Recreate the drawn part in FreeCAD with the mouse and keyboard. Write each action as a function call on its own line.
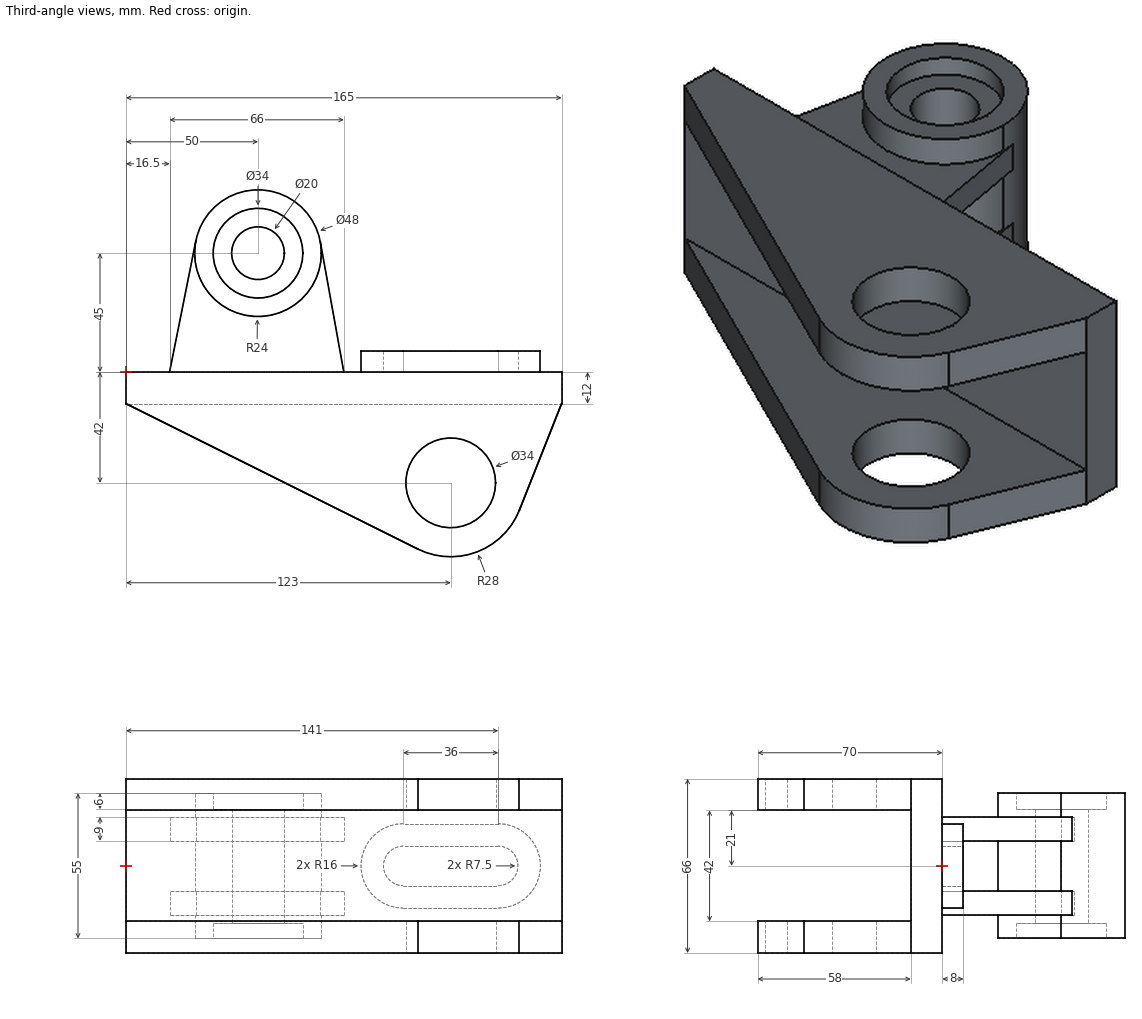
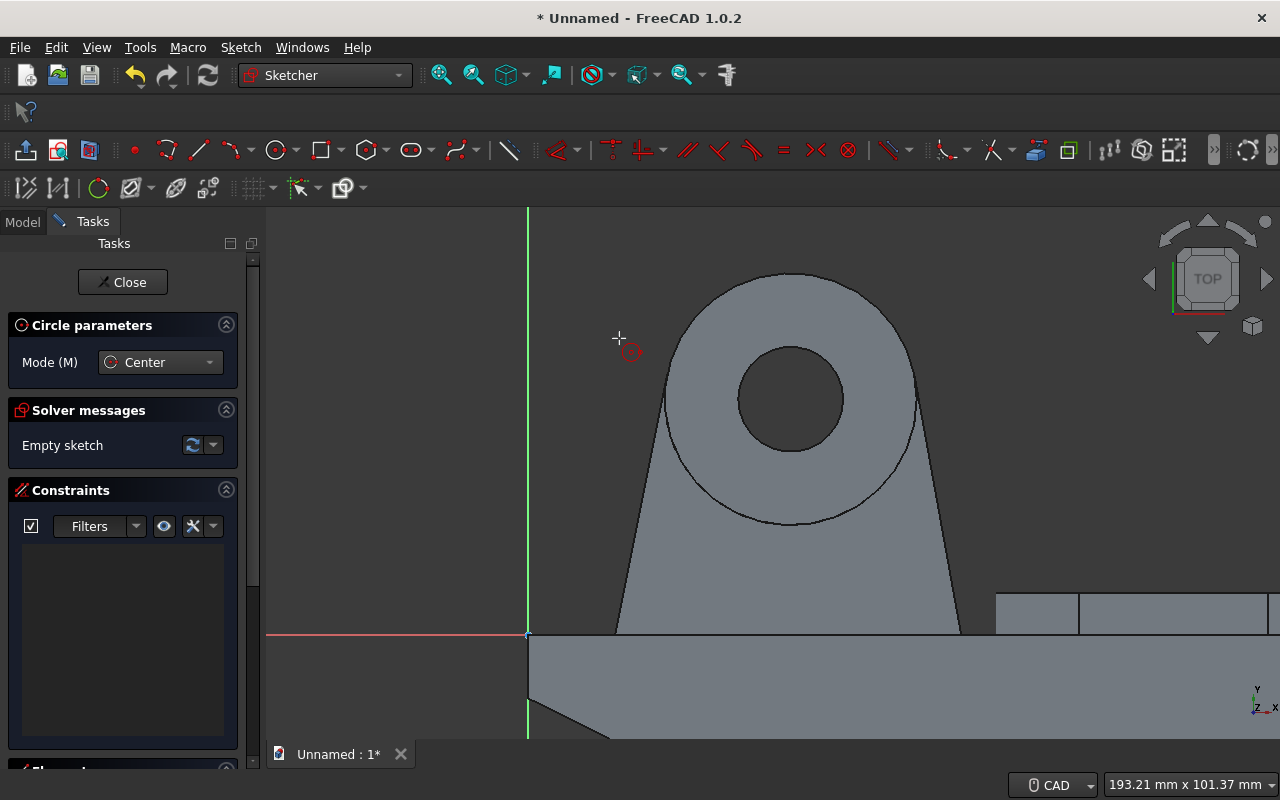
click(791, 399)
move(854, 336)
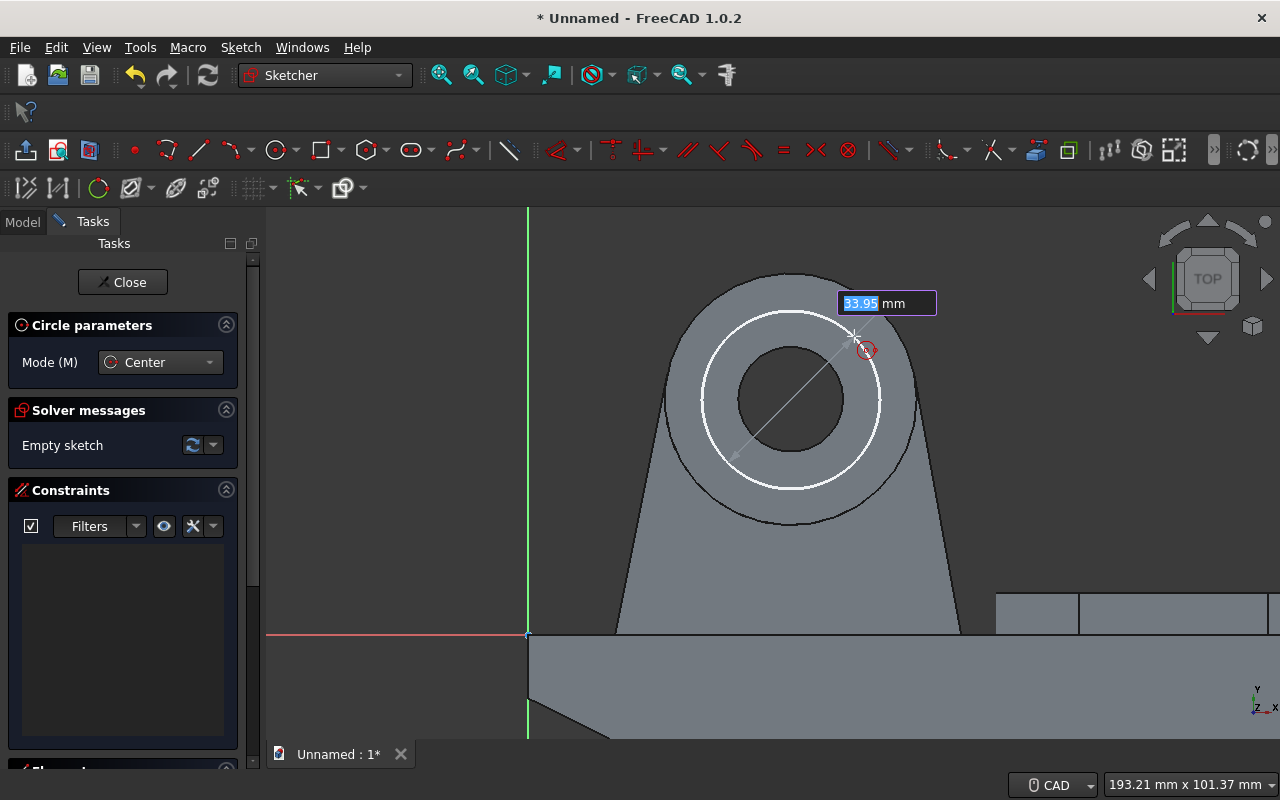
text(34)
key(Return)
key(Escape)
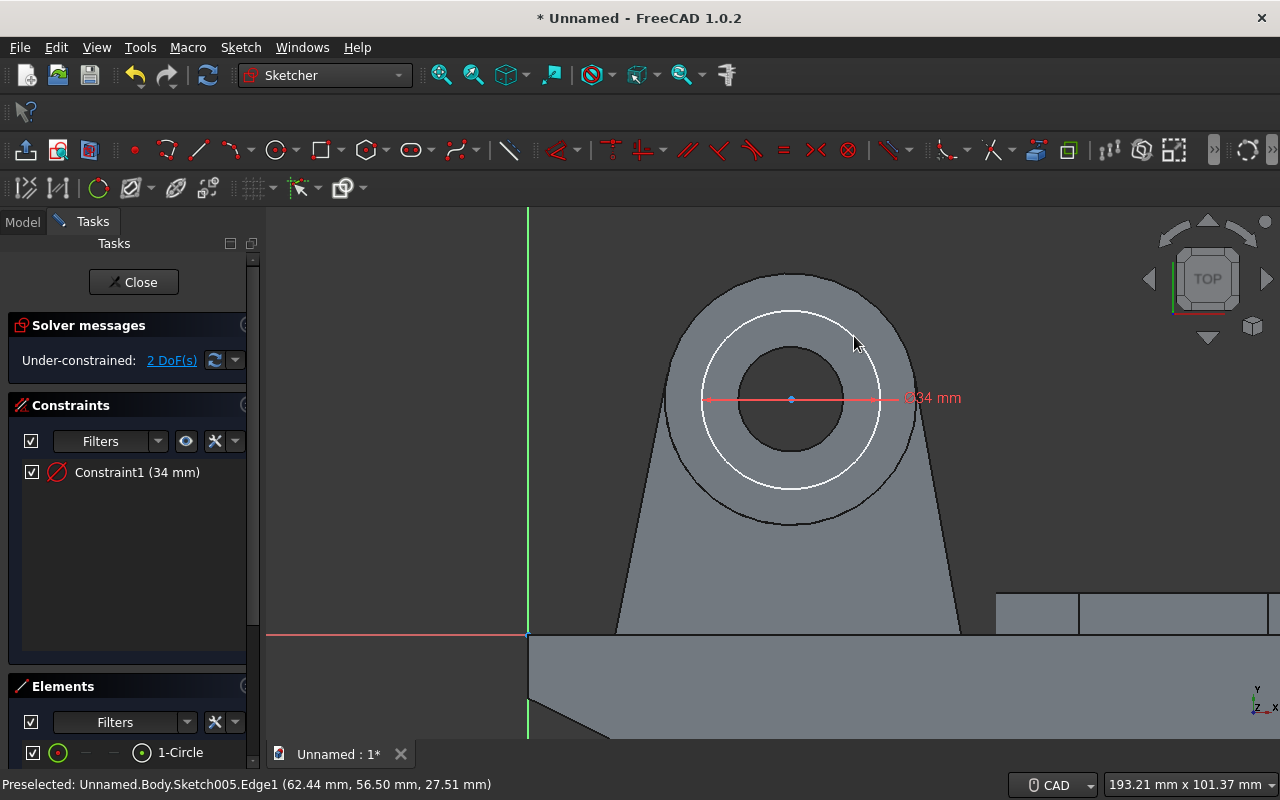
key(d)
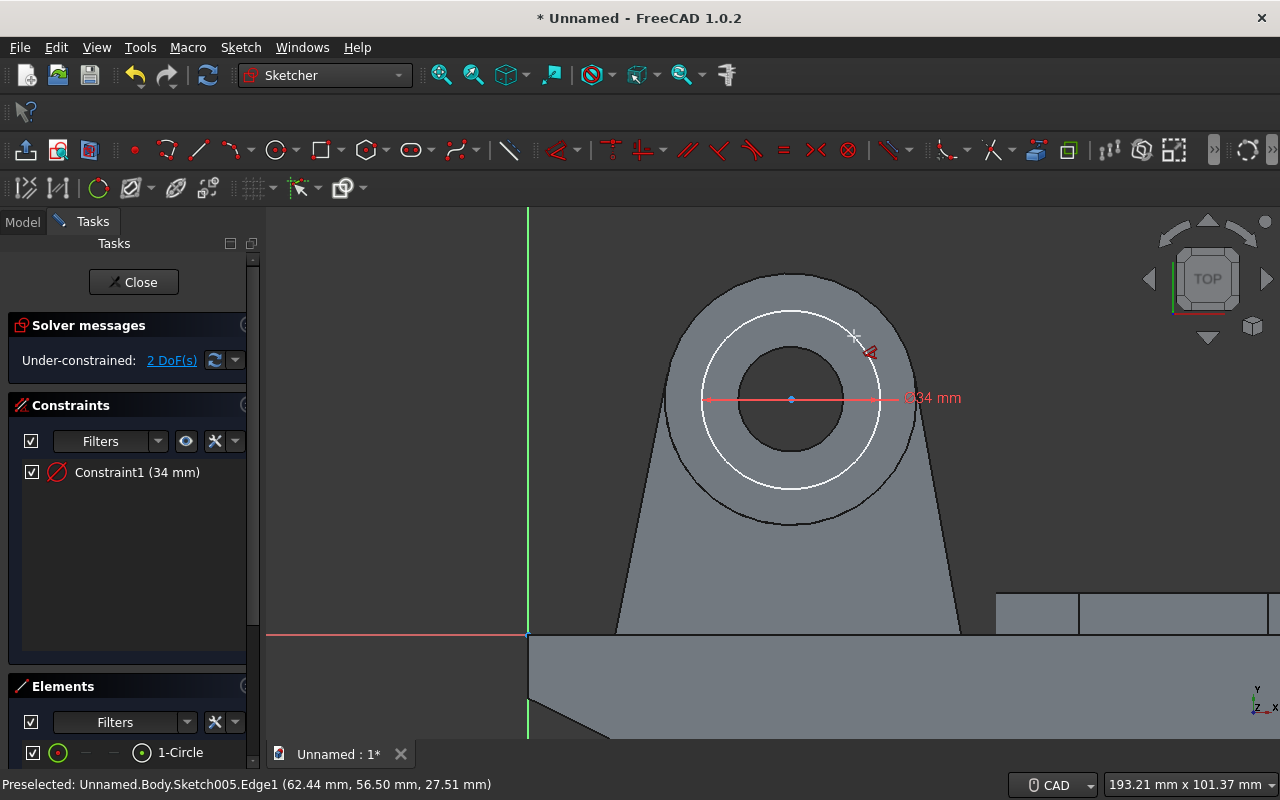
click(791, 400)
click(660, 669)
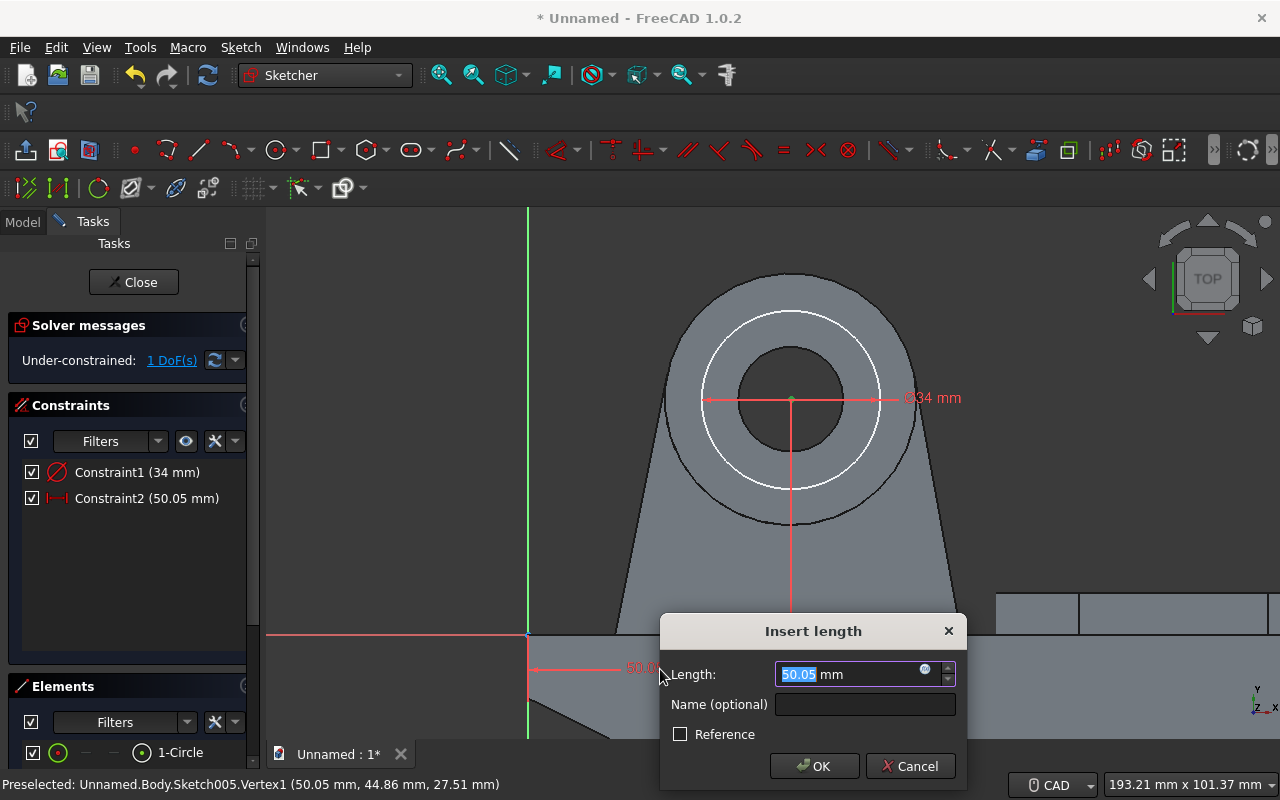
text(50)
key(Return)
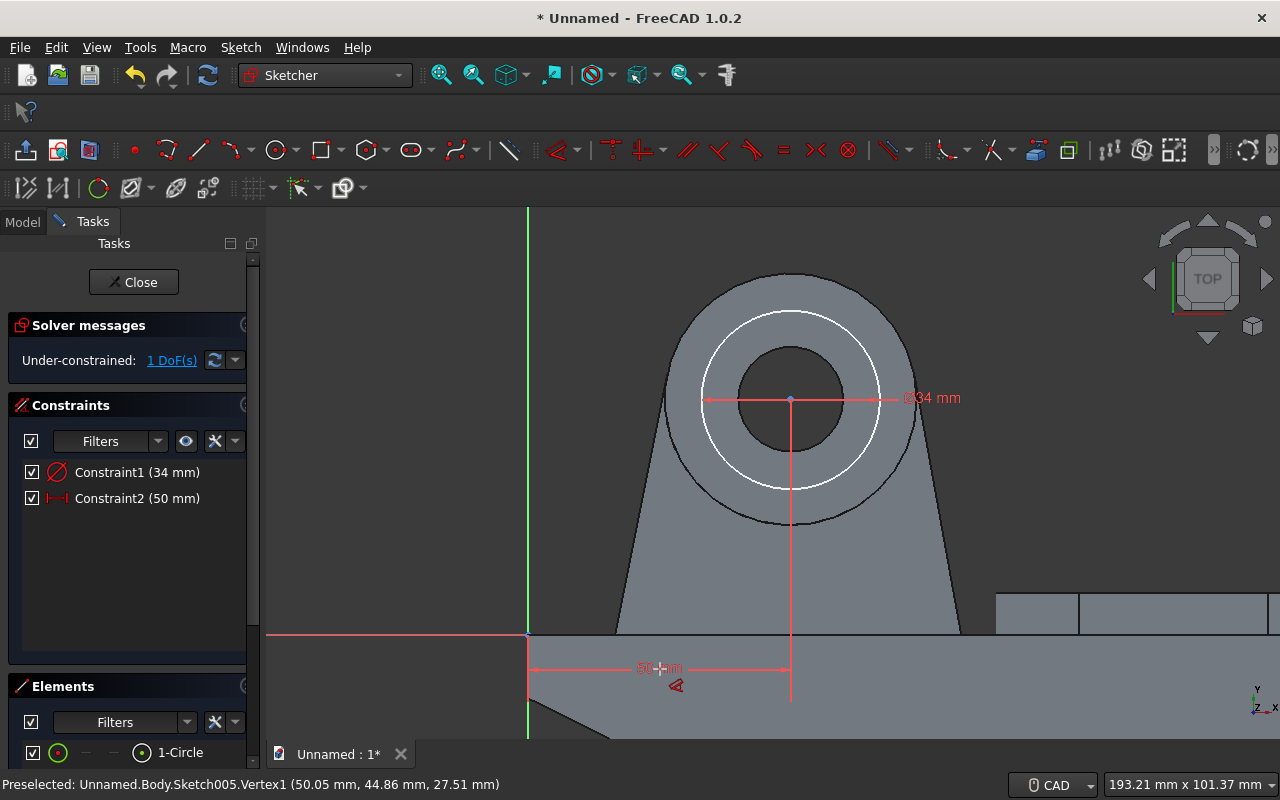
click(791, 400)
click(494, 518)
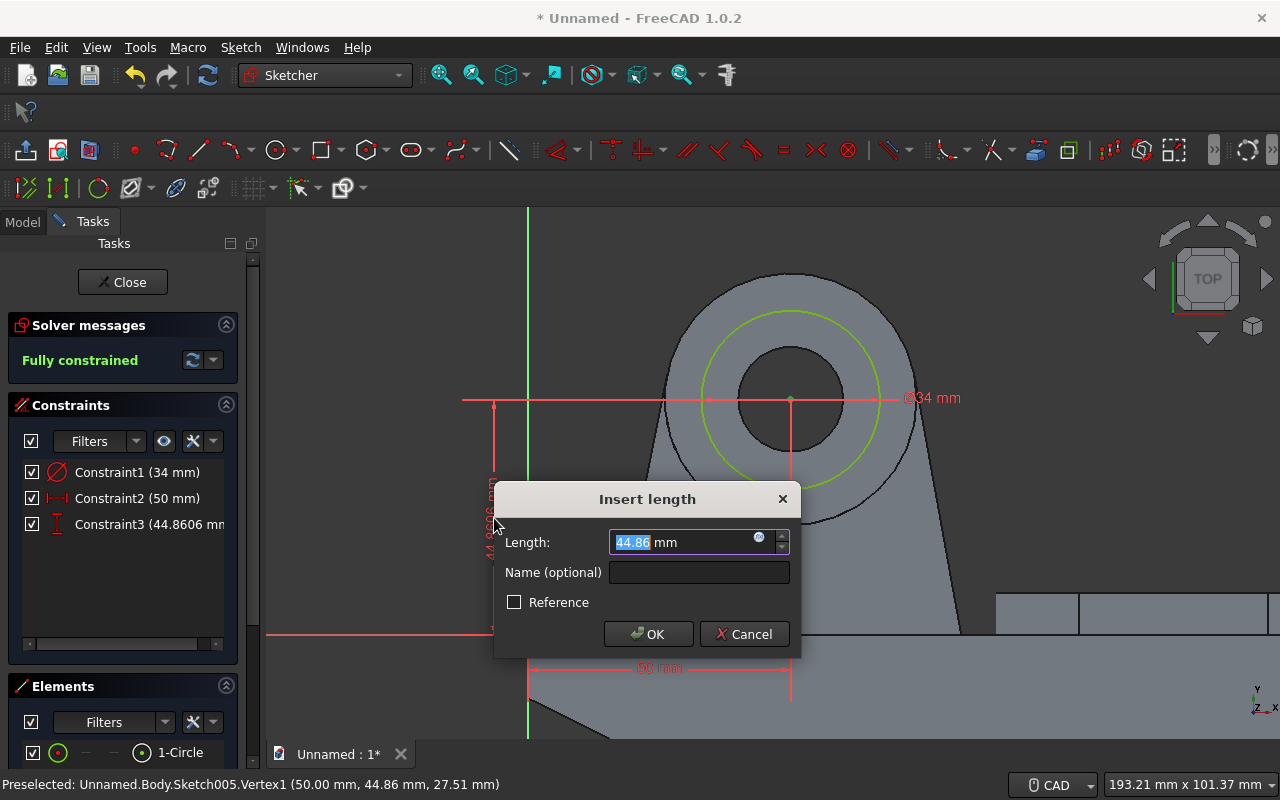
text(45)
key(Return)
key(Escape)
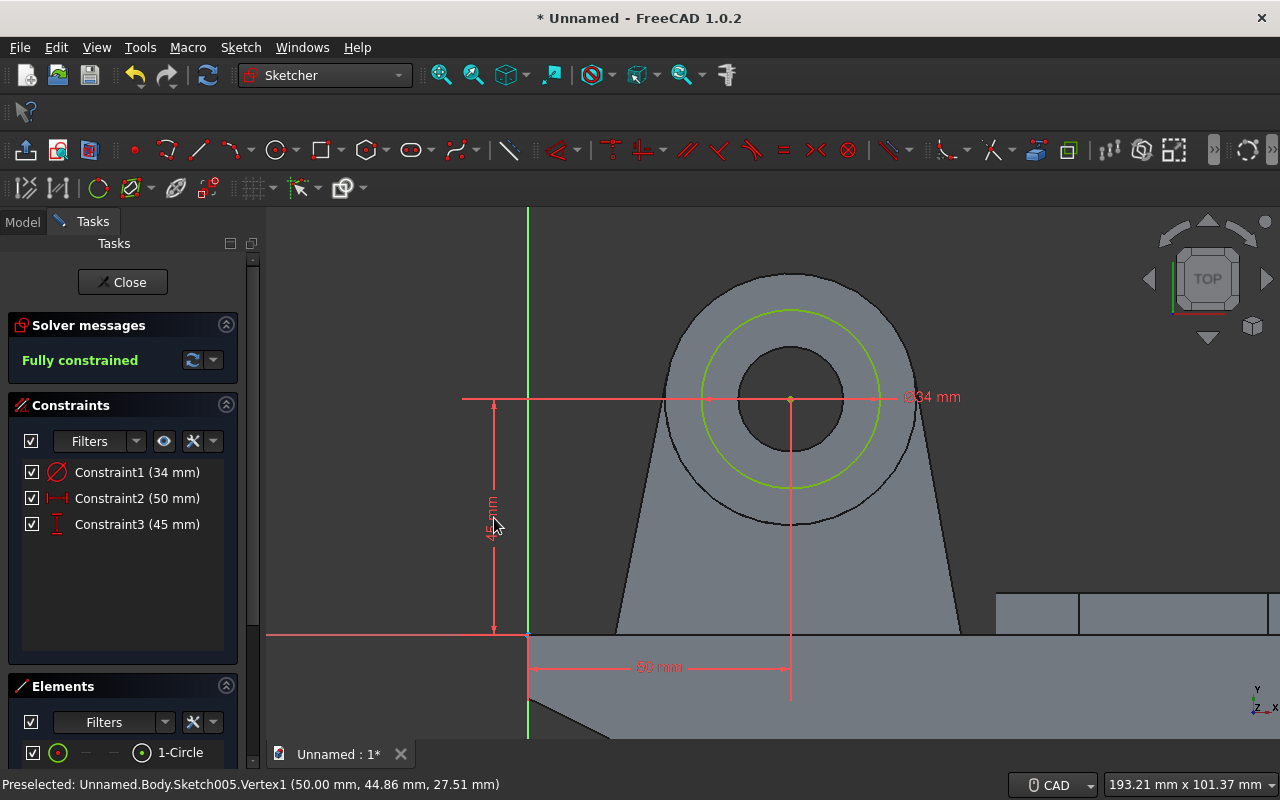
click(123, 282)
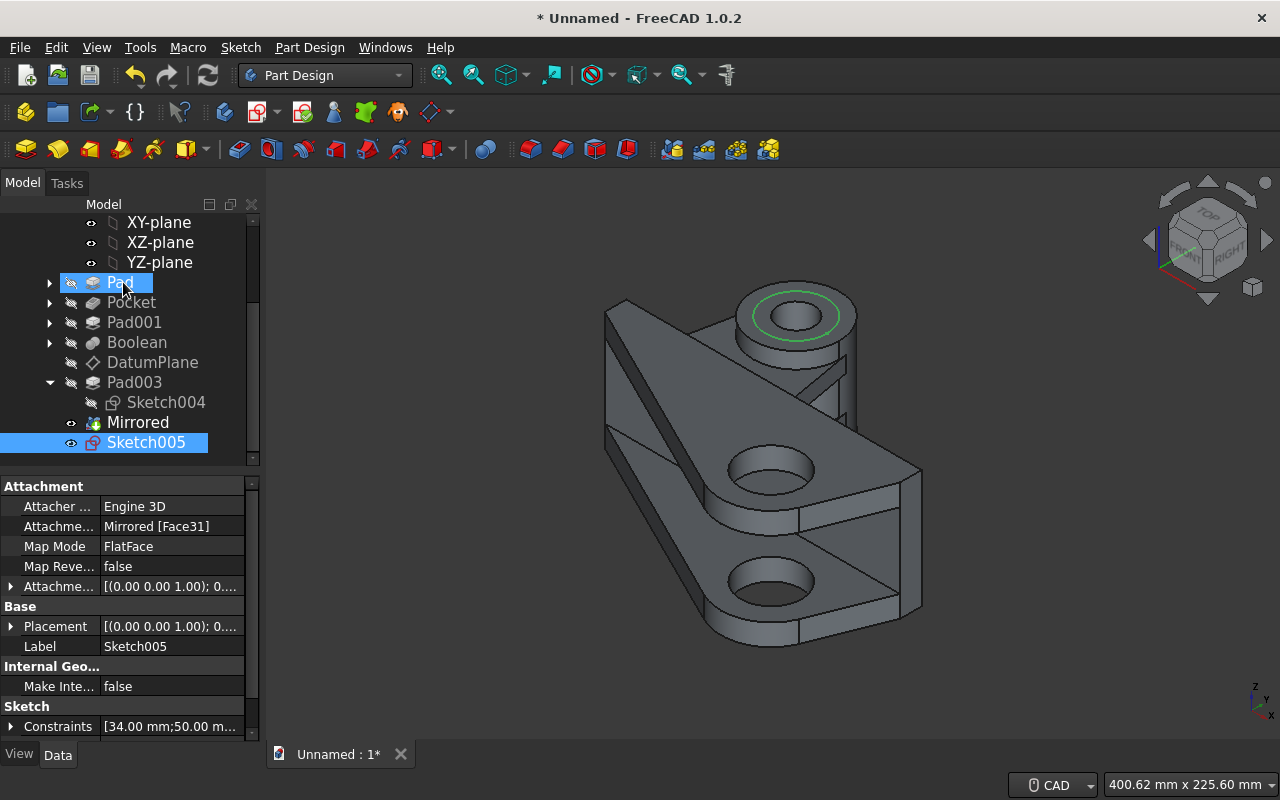
click(240, 150)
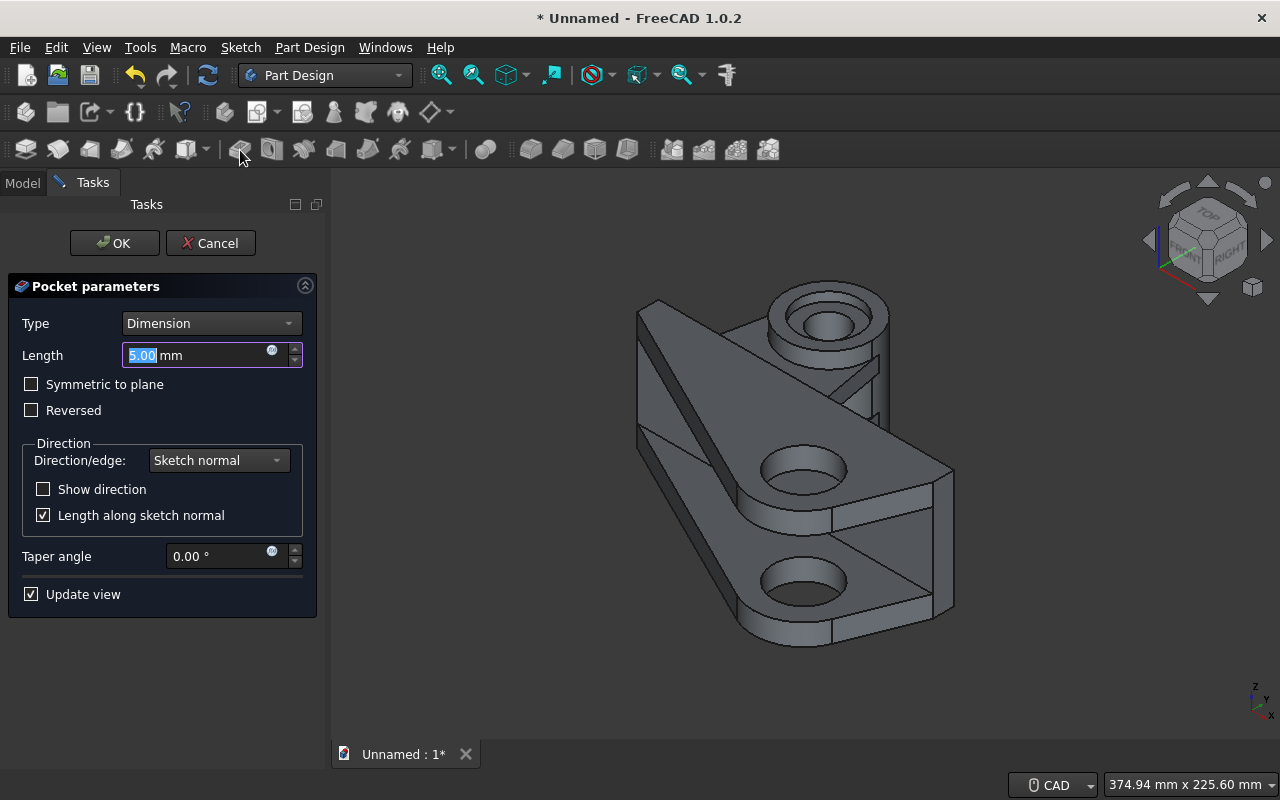
text(6)
key(Tab)